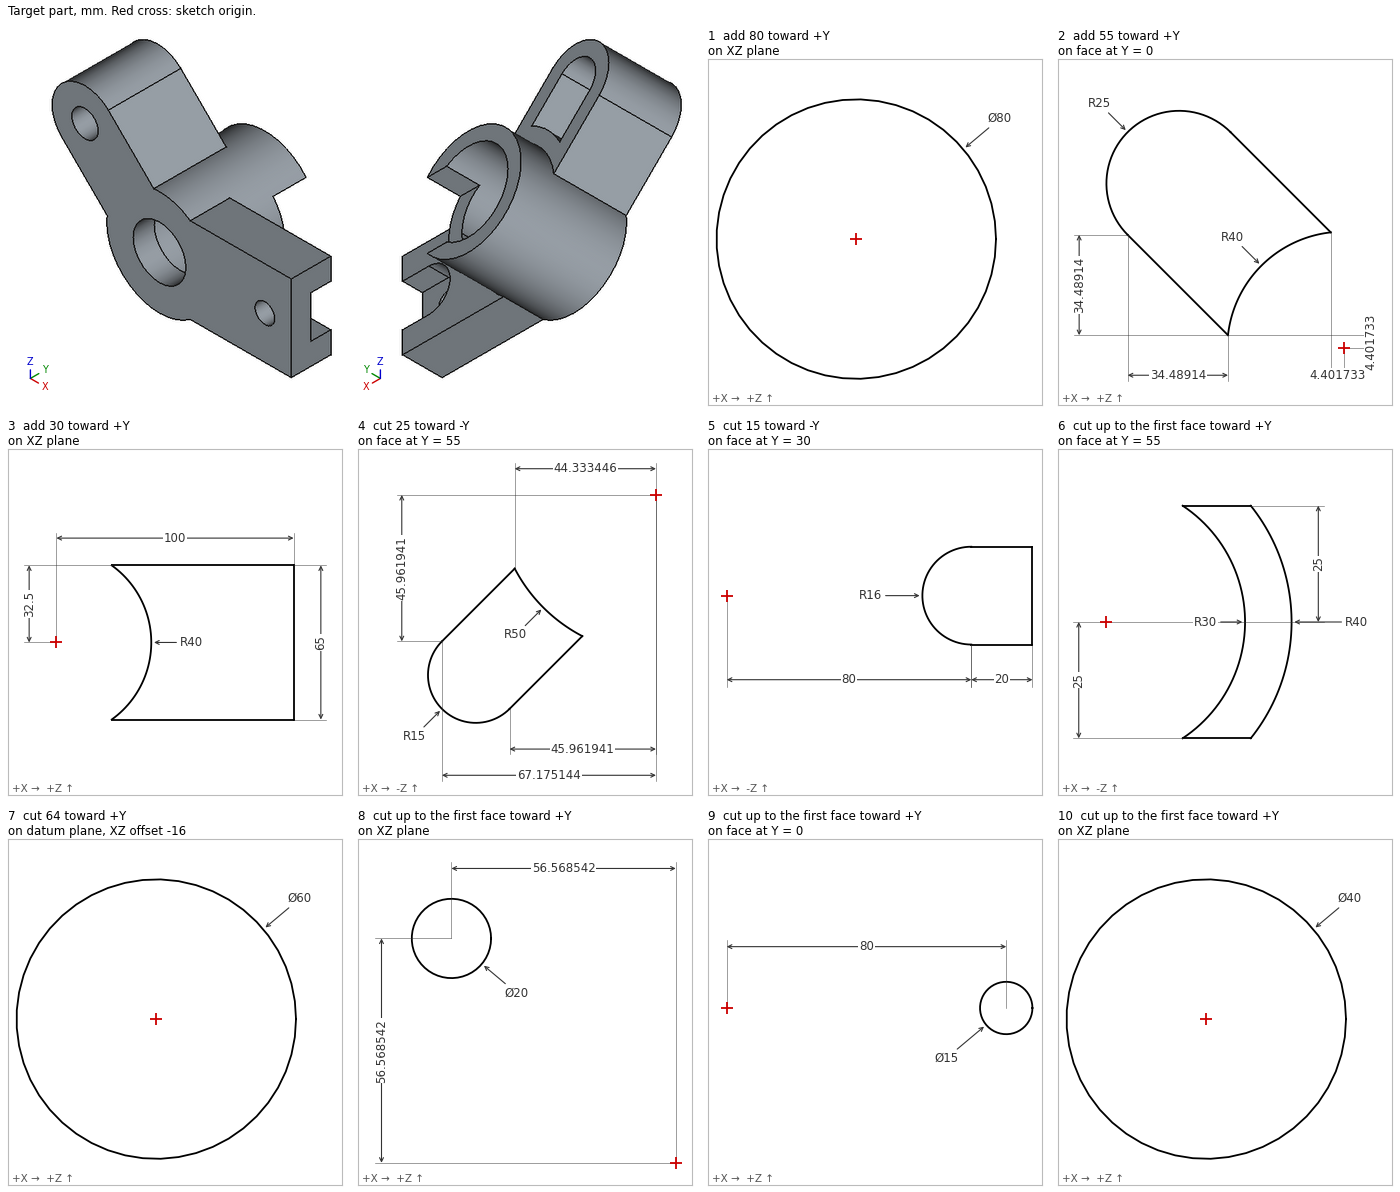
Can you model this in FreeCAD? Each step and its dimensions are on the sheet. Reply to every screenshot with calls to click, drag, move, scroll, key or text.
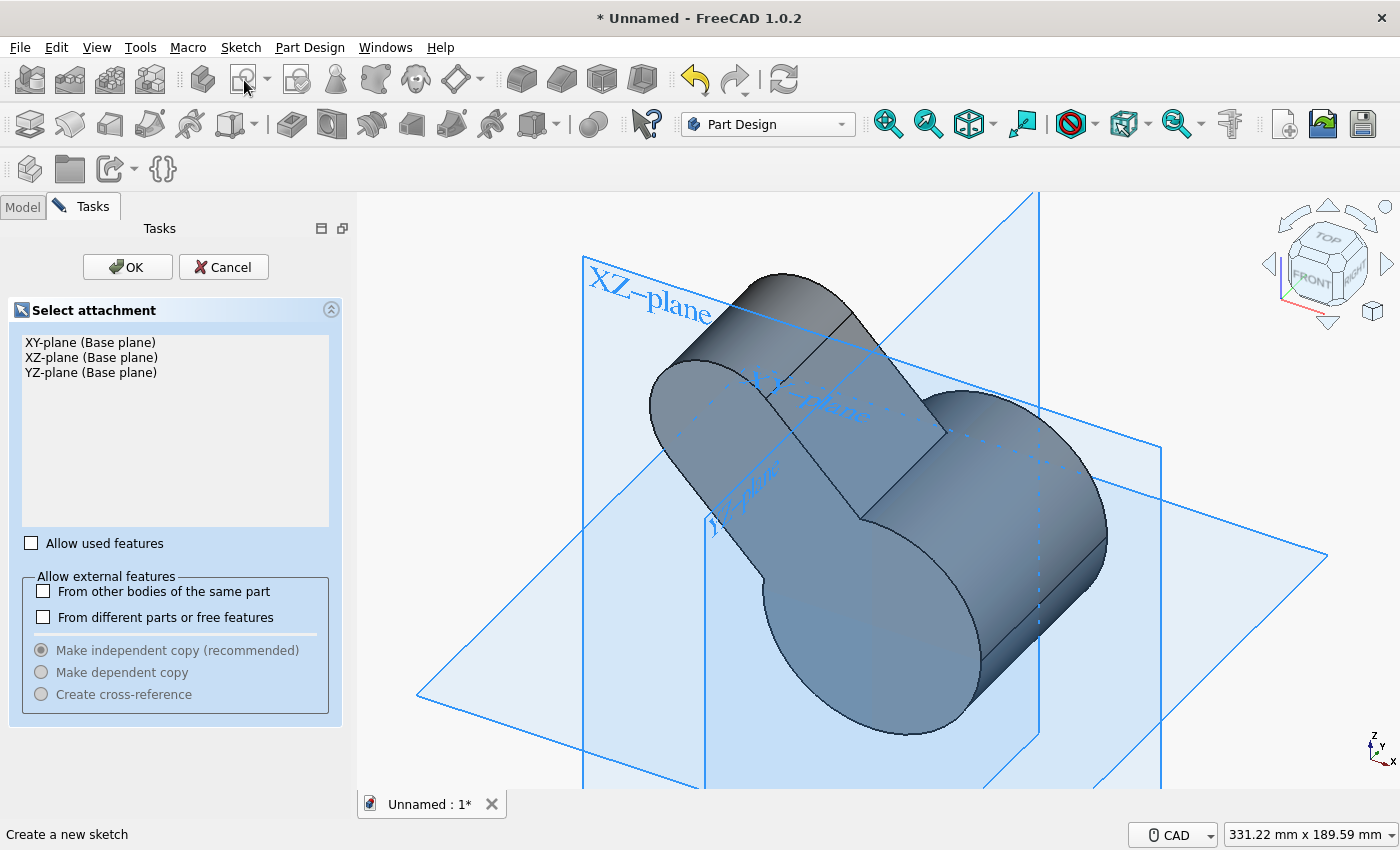
click(82, 358)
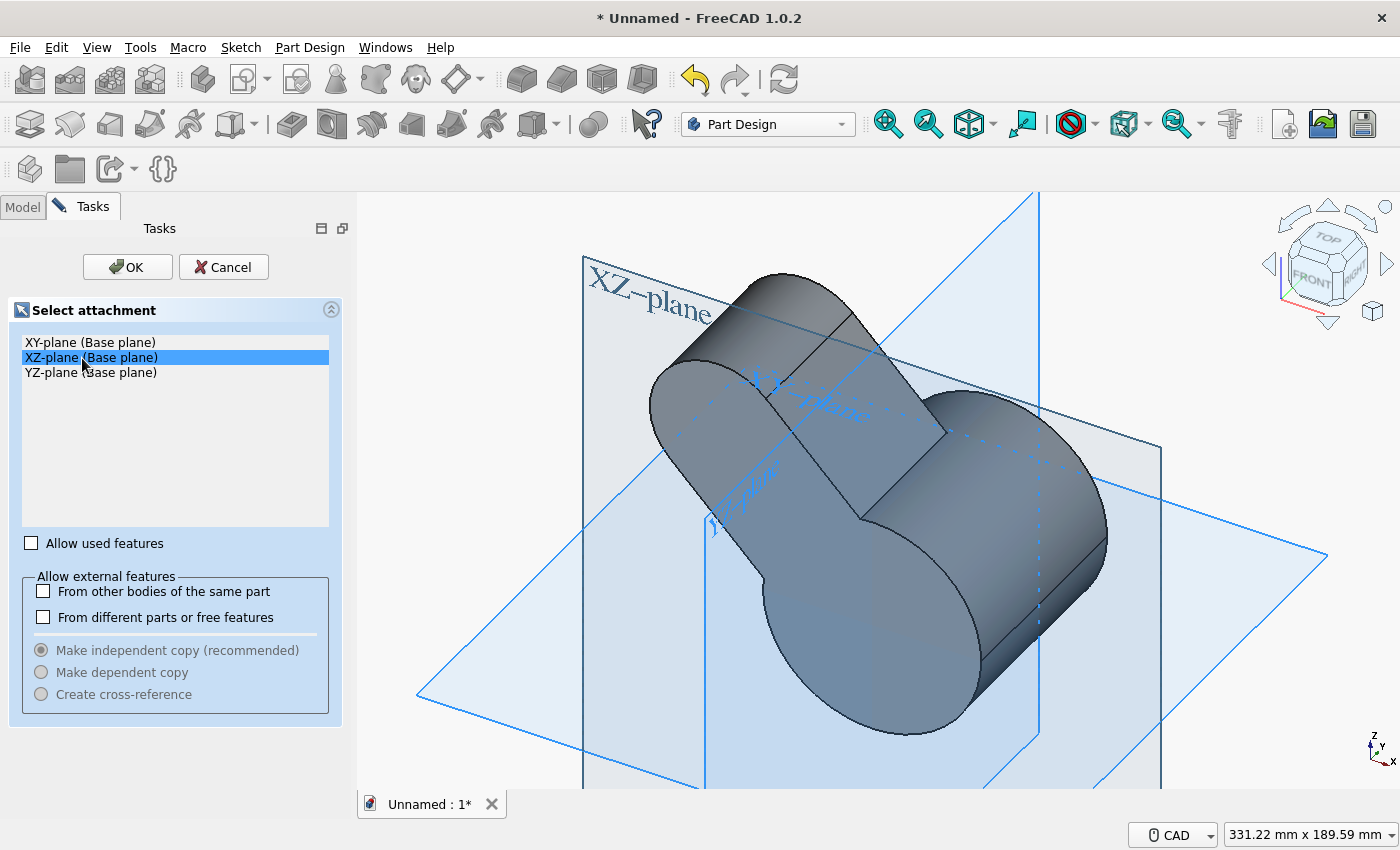
click(128, 267)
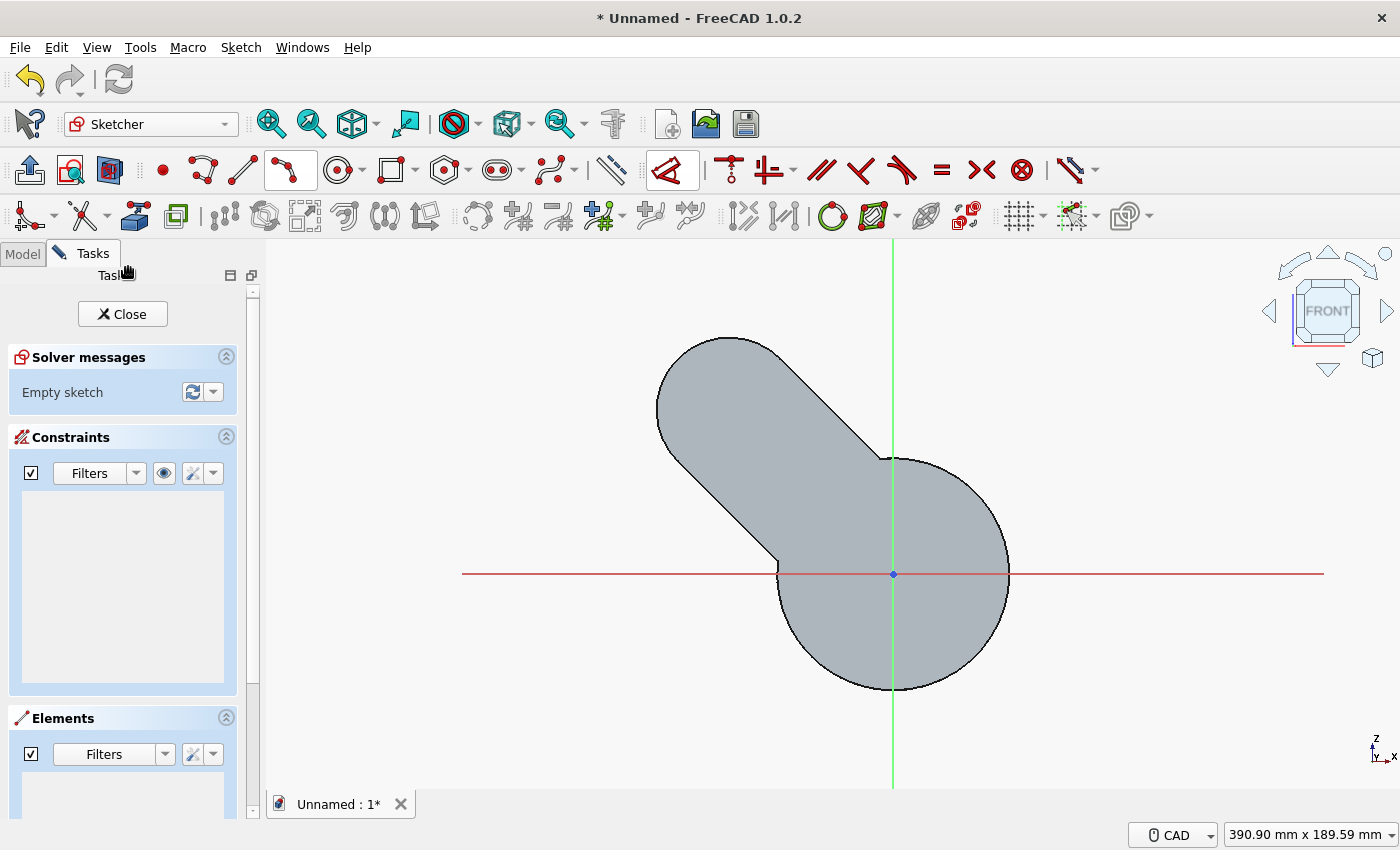
scroll(1235, 648, up, 3)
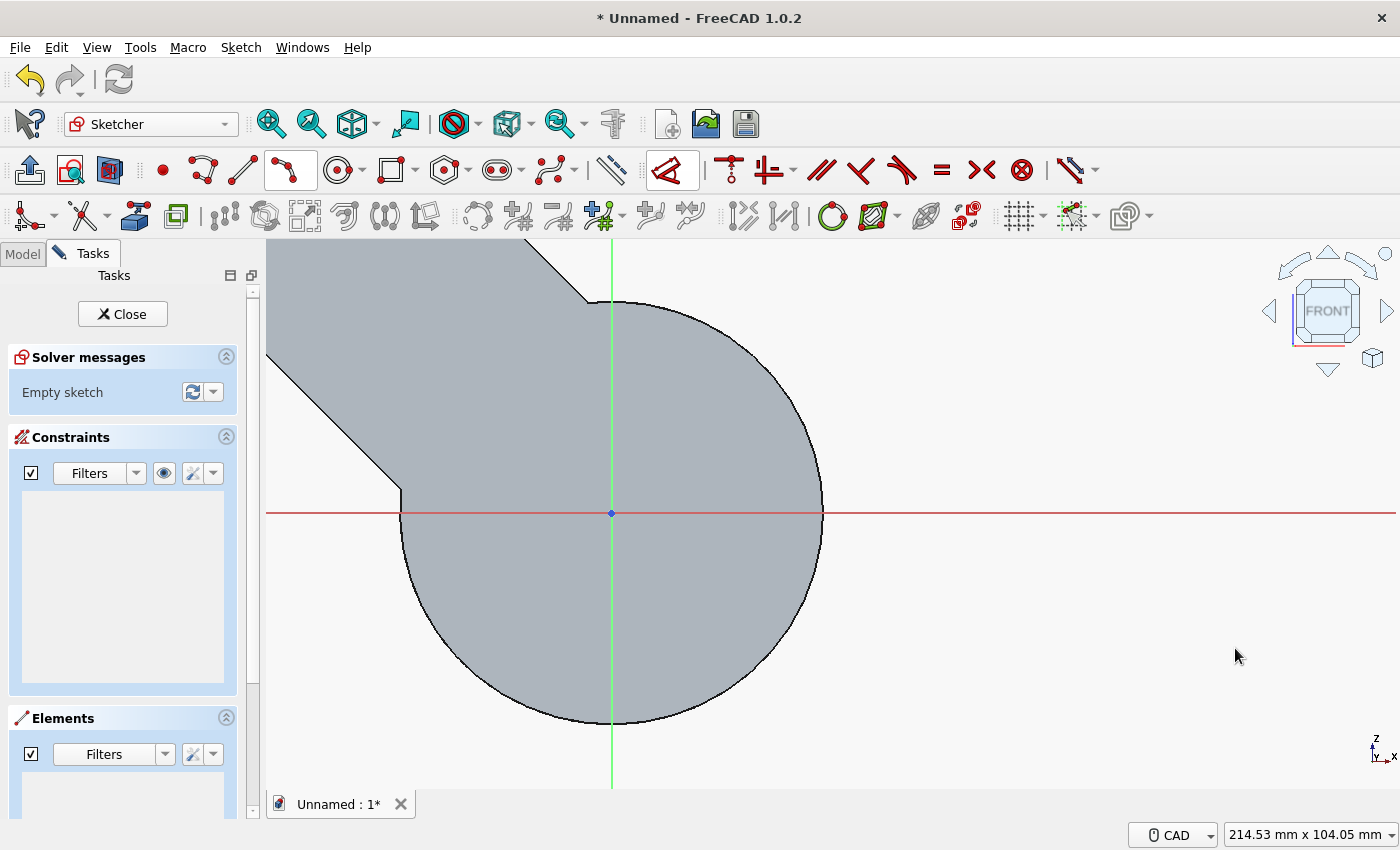
click(204, 170)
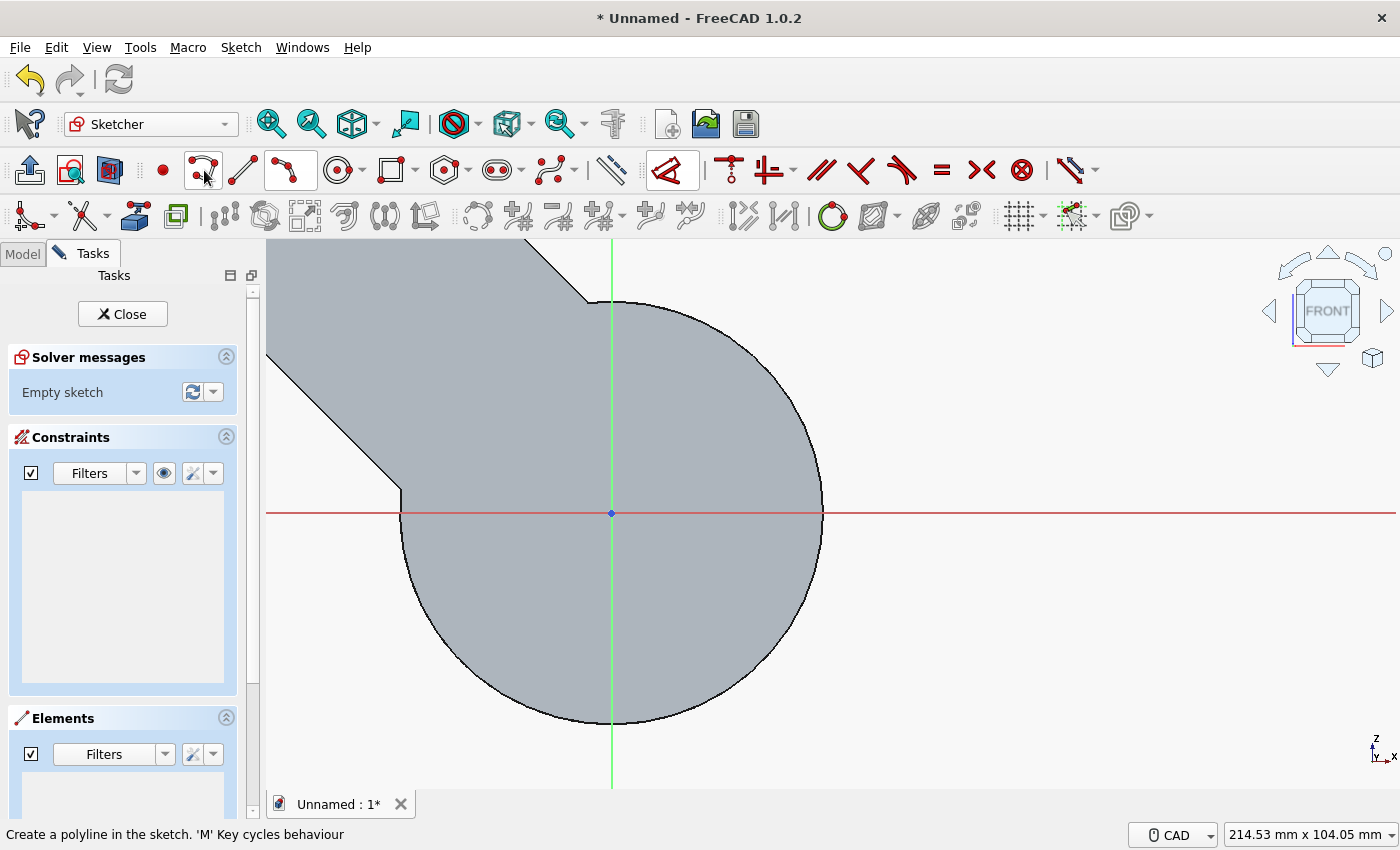
click(735, 341)
click(1140, 341)
click(1140, 685)
click(735, 685)
right_click(735, 685)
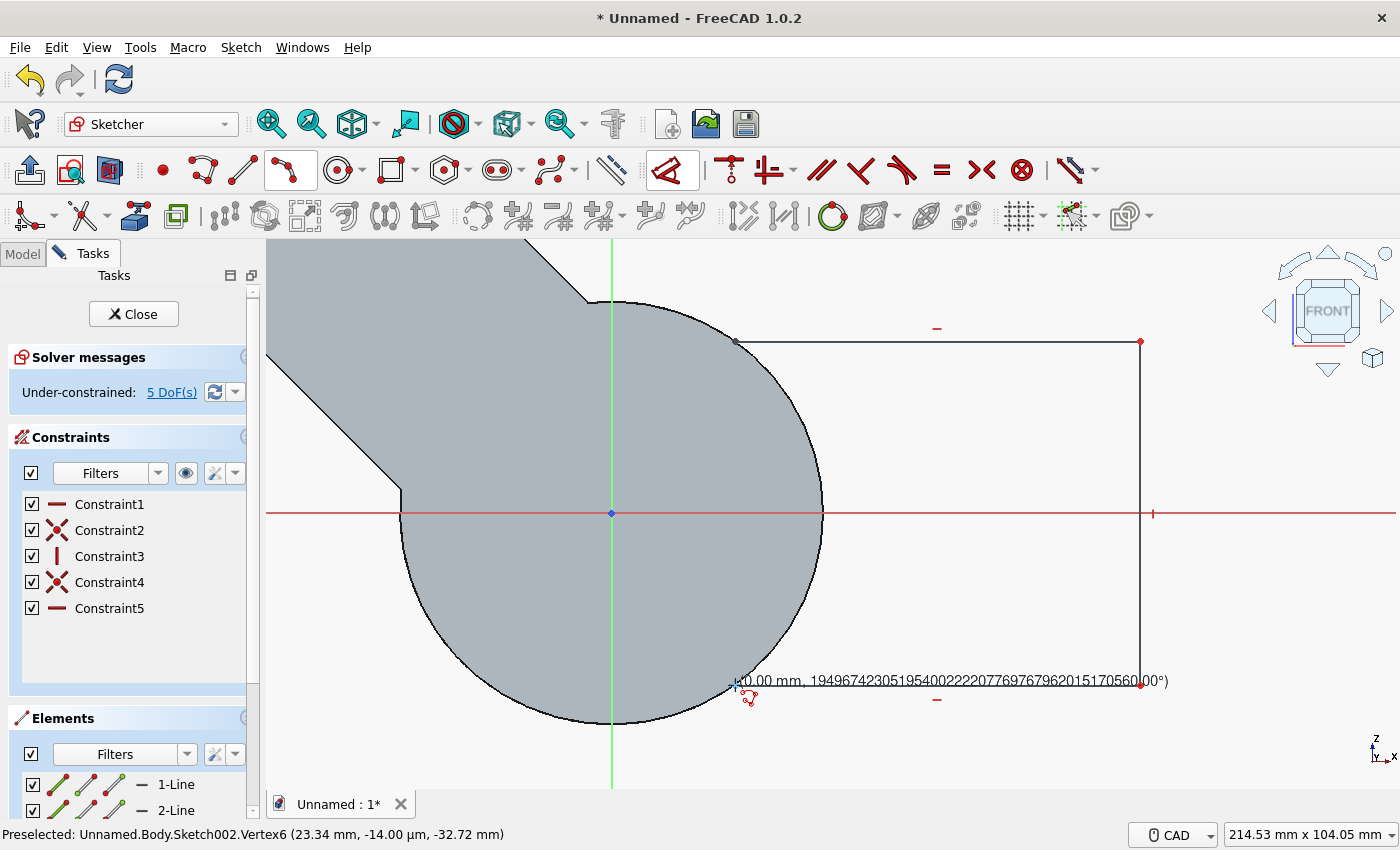
click(284, 170)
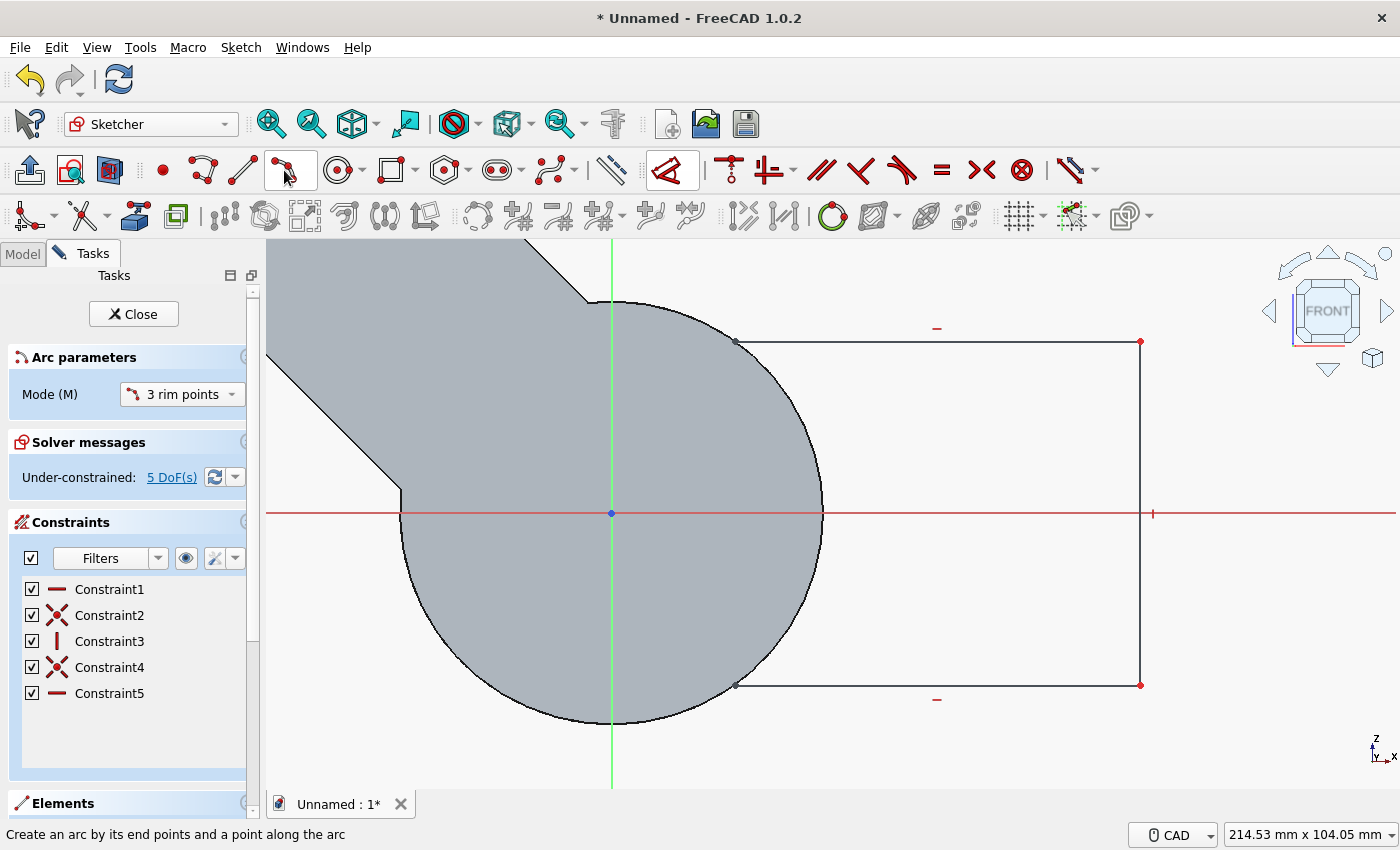
click(735, 686)
click(735, 342)
click(819, 553)
key(Escape)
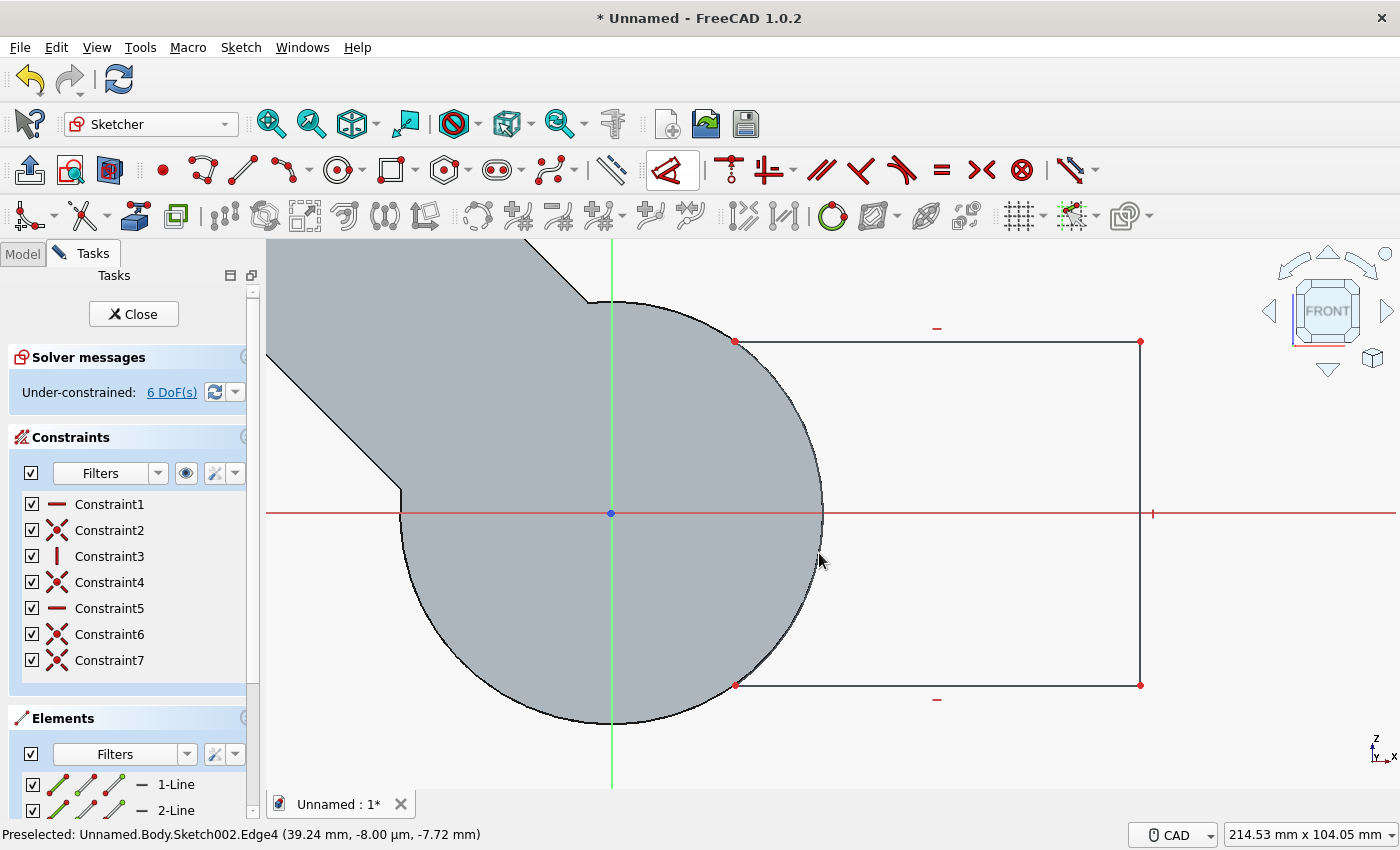
drag(600, 503, 622, 524)